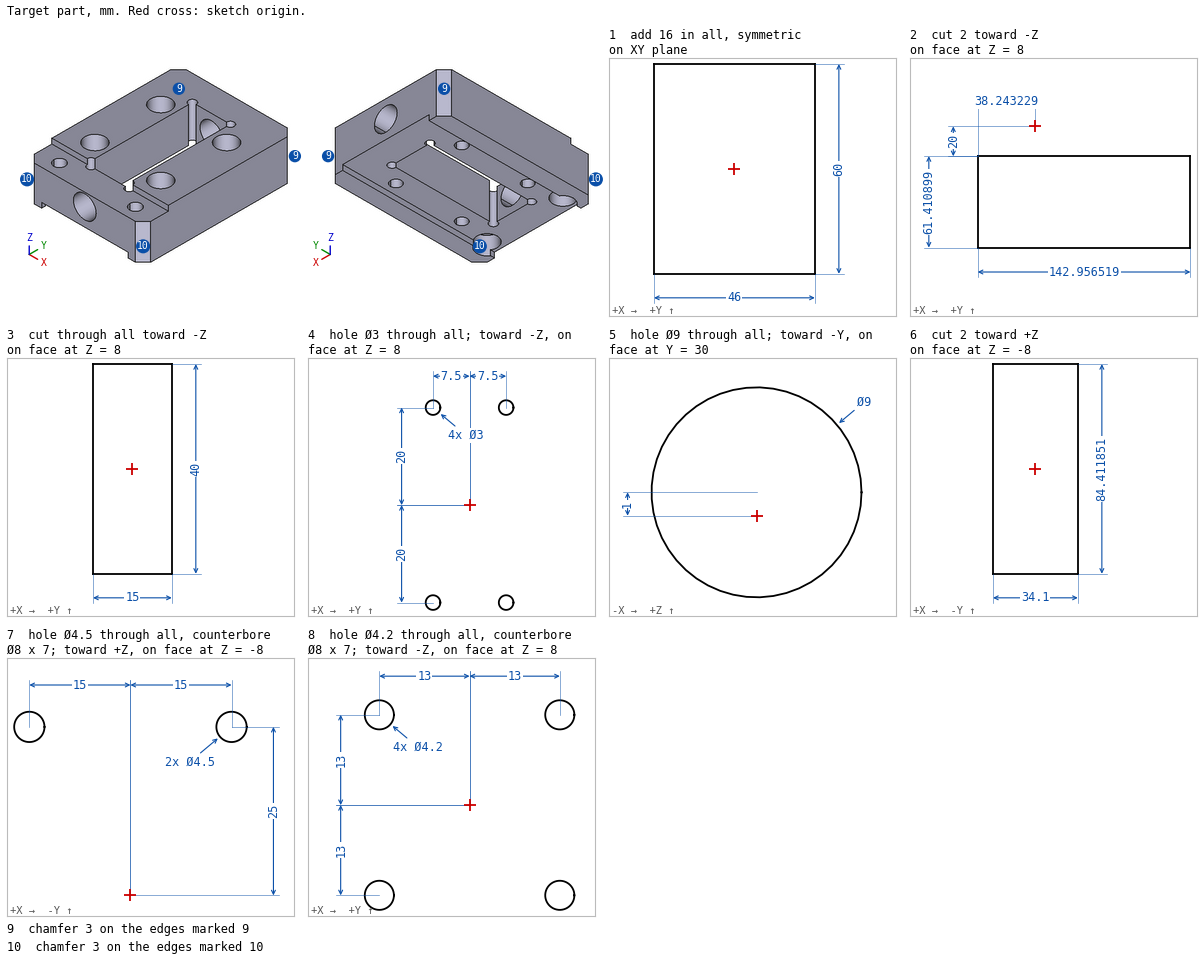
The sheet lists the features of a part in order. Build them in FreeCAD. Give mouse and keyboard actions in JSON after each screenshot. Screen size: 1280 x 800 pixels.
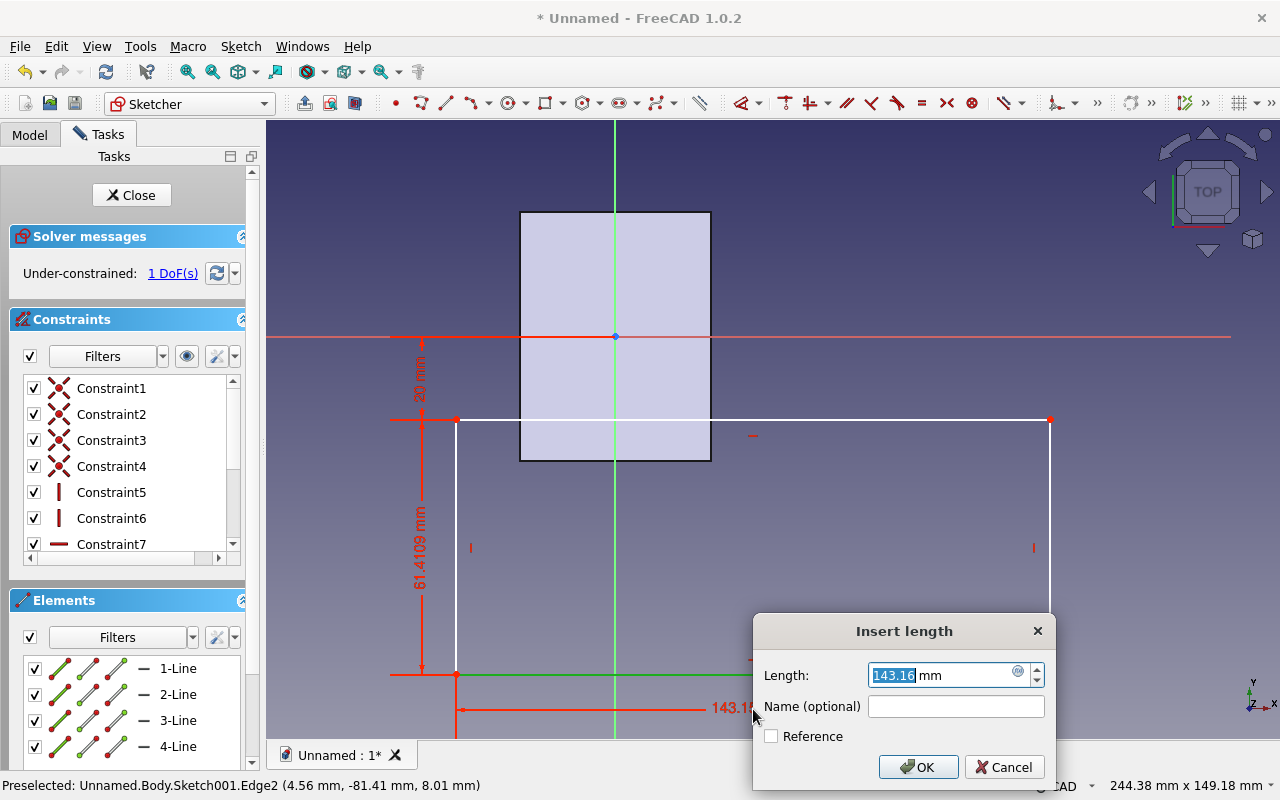
{"action": "type", "text": "142.956519"}
{"action": "key", "text": "Return"}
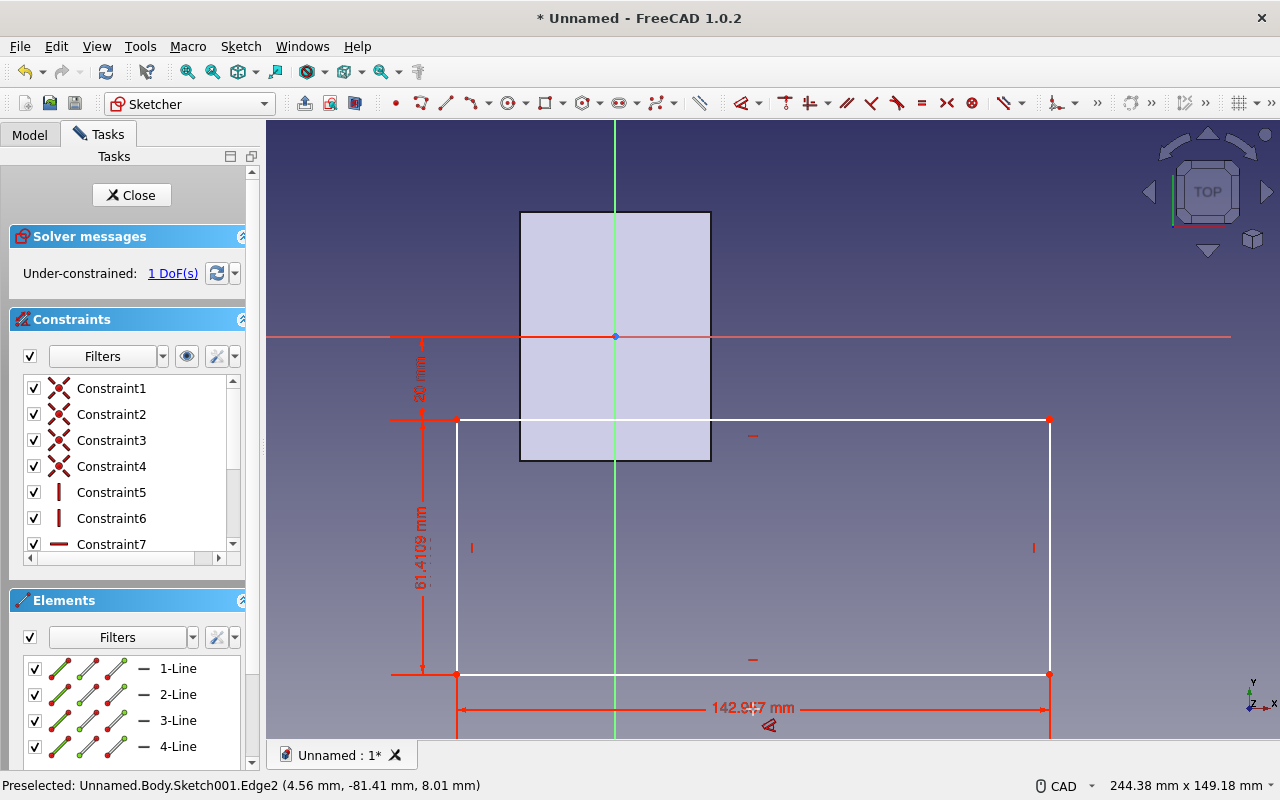
{"action": "left_click", "coordinate": [457, 420]}
{"action": "left_click", "coordinate": [536, 303]}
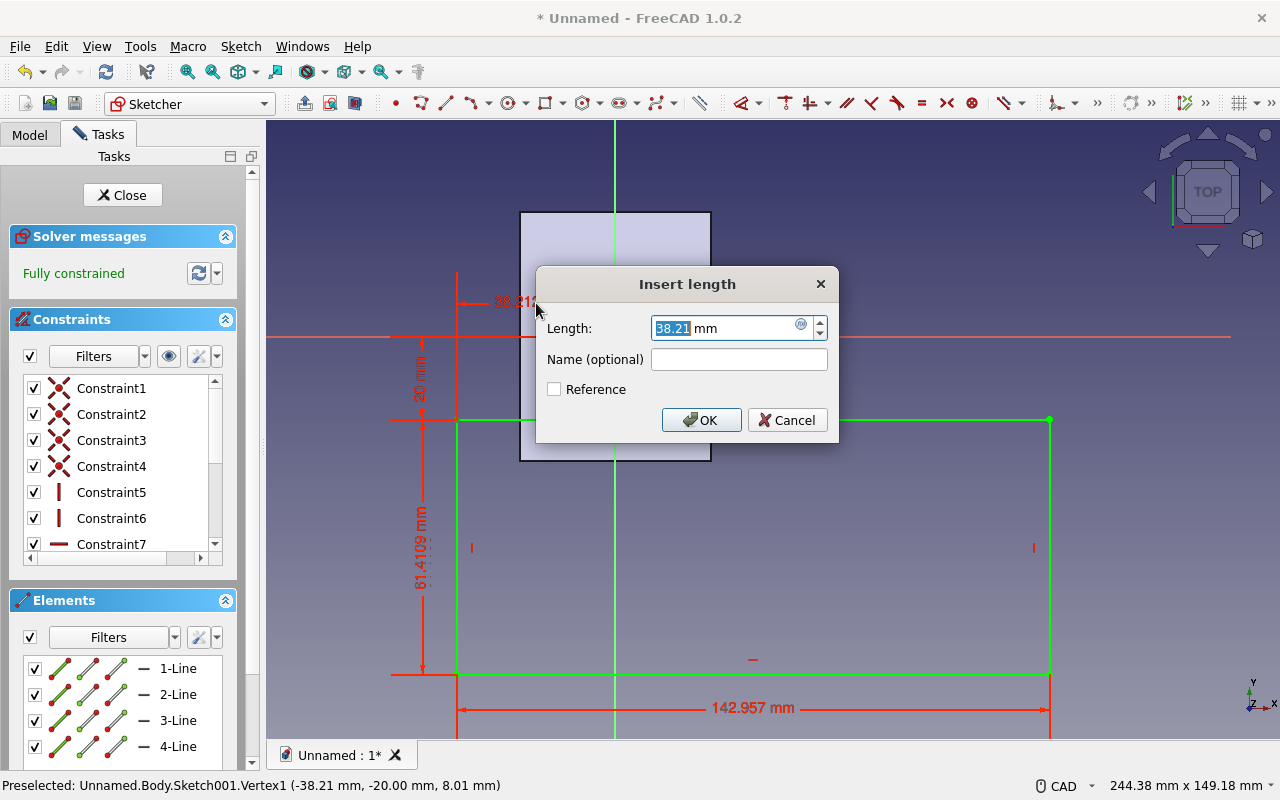
{"action": "type", "text": "38.243229"}
{"action": "key", "text": "Return"}
{"action": "key", "text": "Escape"}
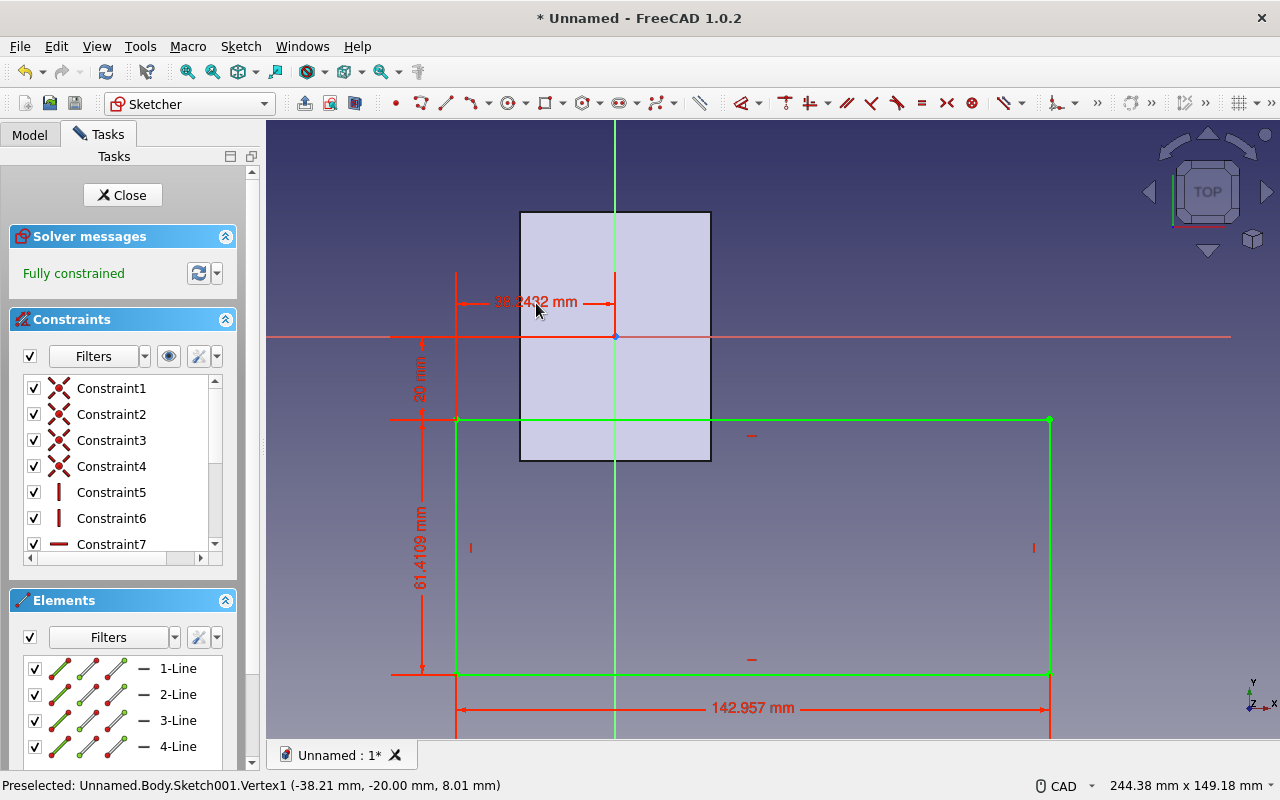
{"action": "left_click", "coordinate": [123, 195]}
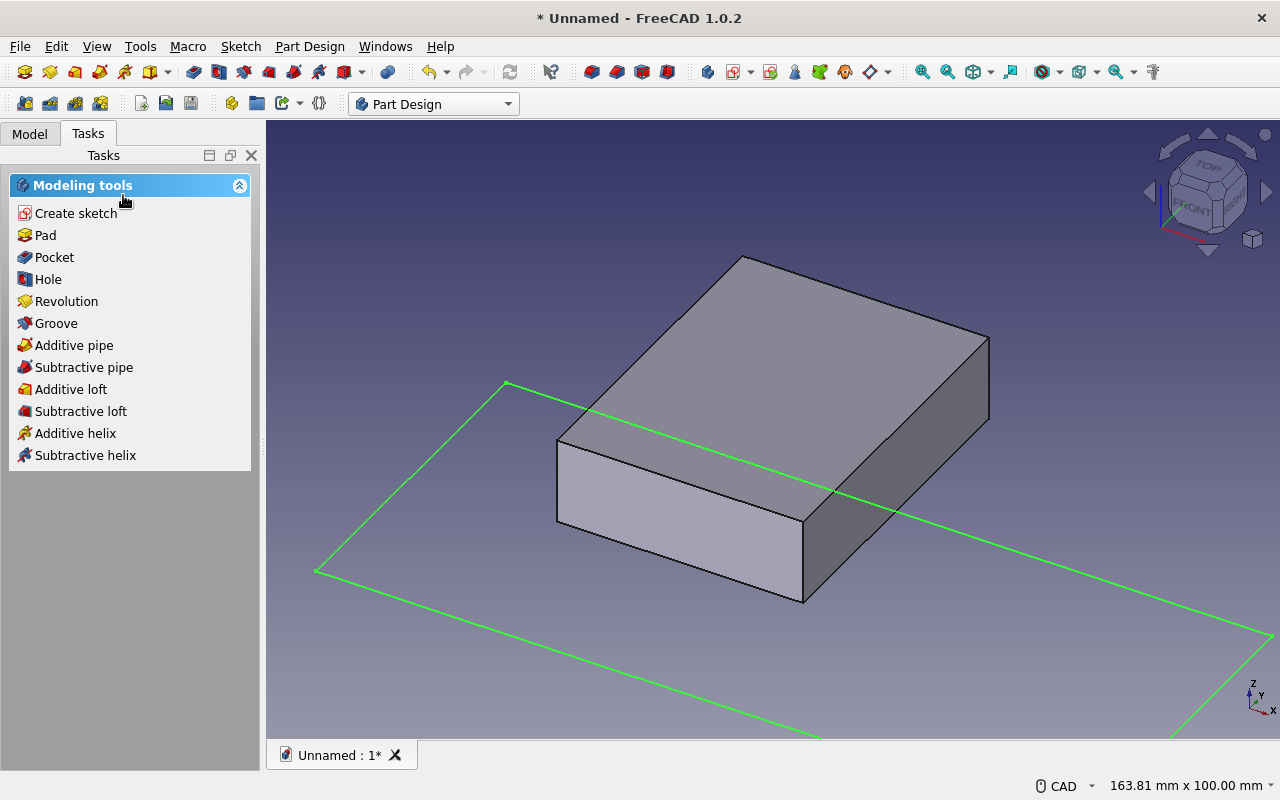
{"action": "left_click", "coordinate": [194, 72]}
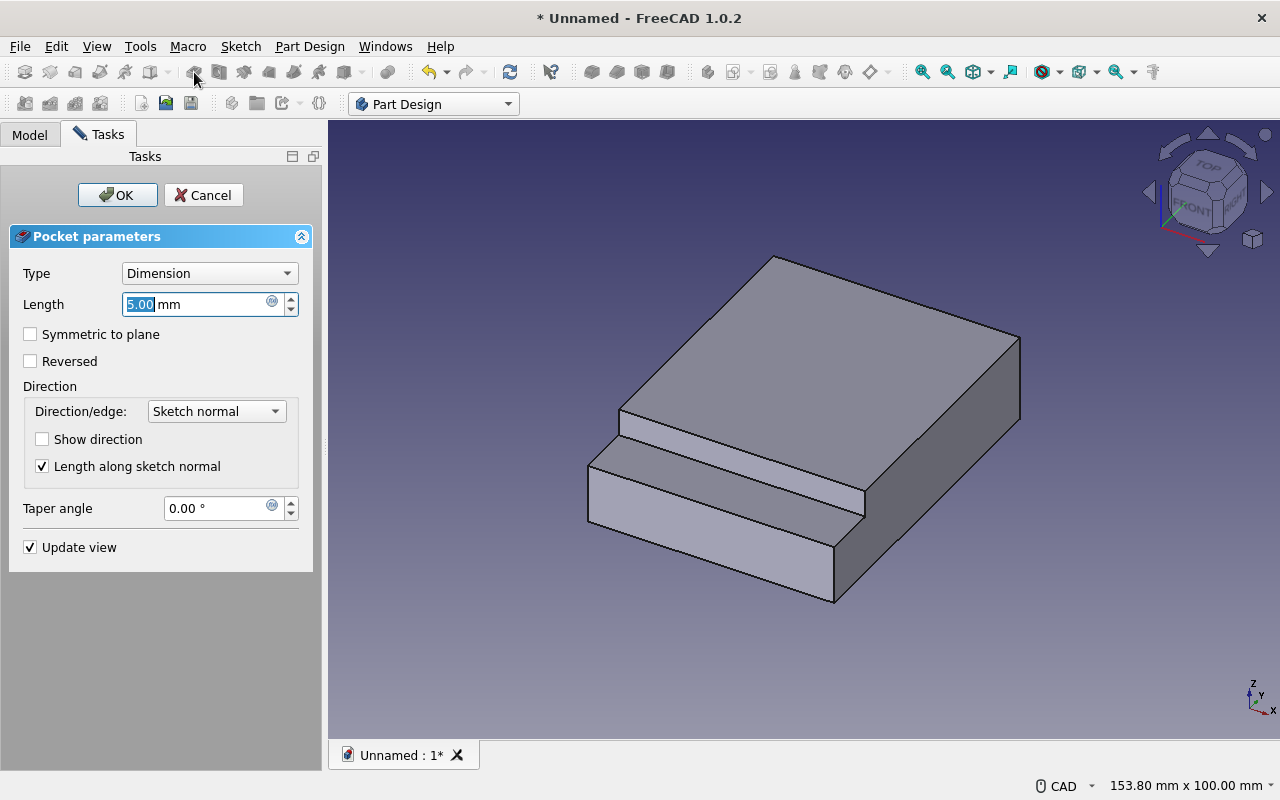
{"action": "type", "text": "2"}
{"action": "key", "text": "Tab"}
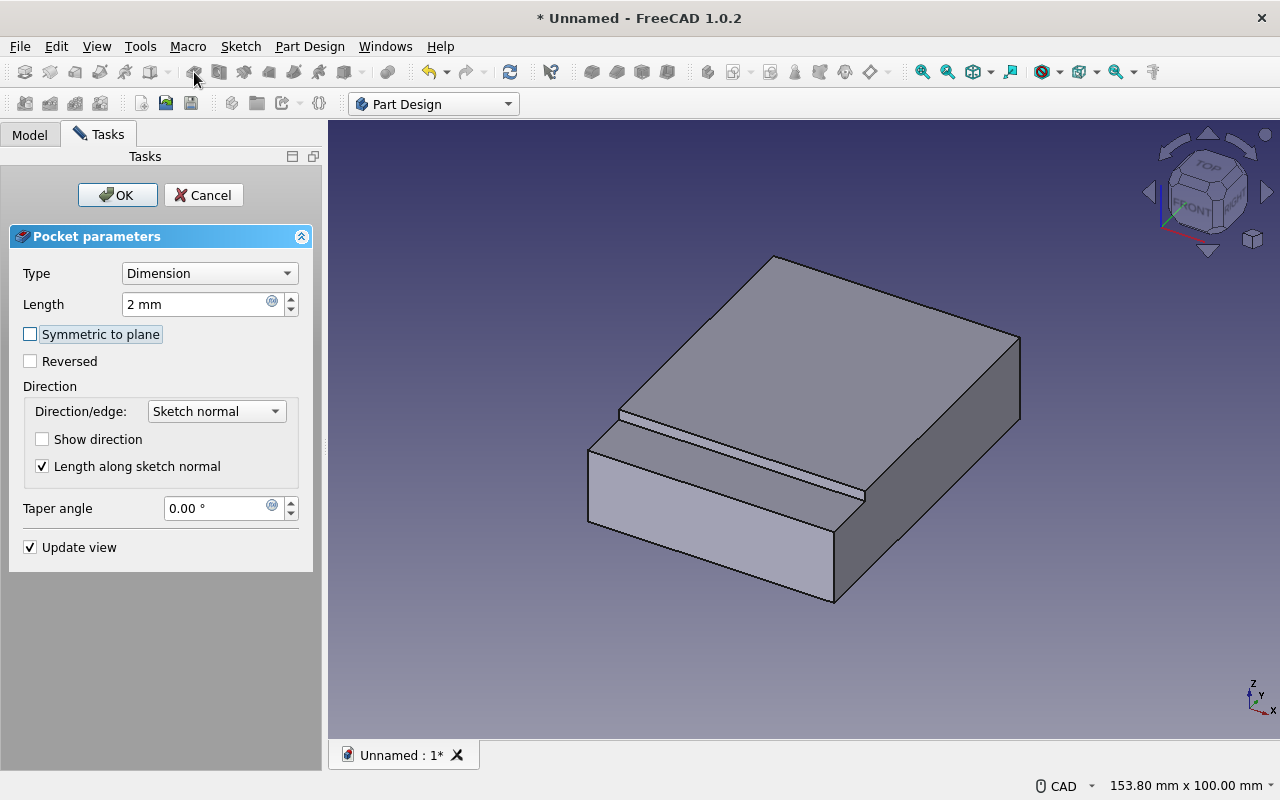
{"action": "left_click", "coordinate": [118, 195]}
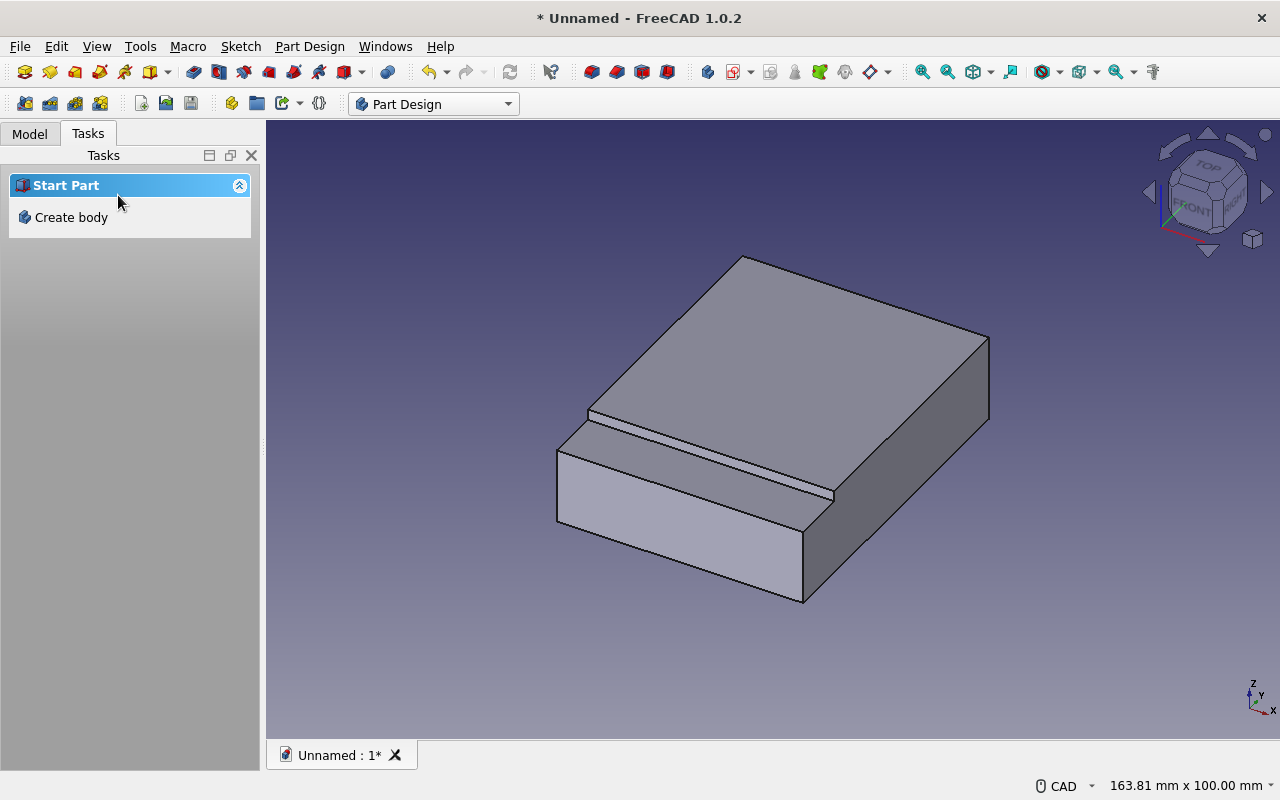
{"action": "left_click", "coordinate": [788, 373]}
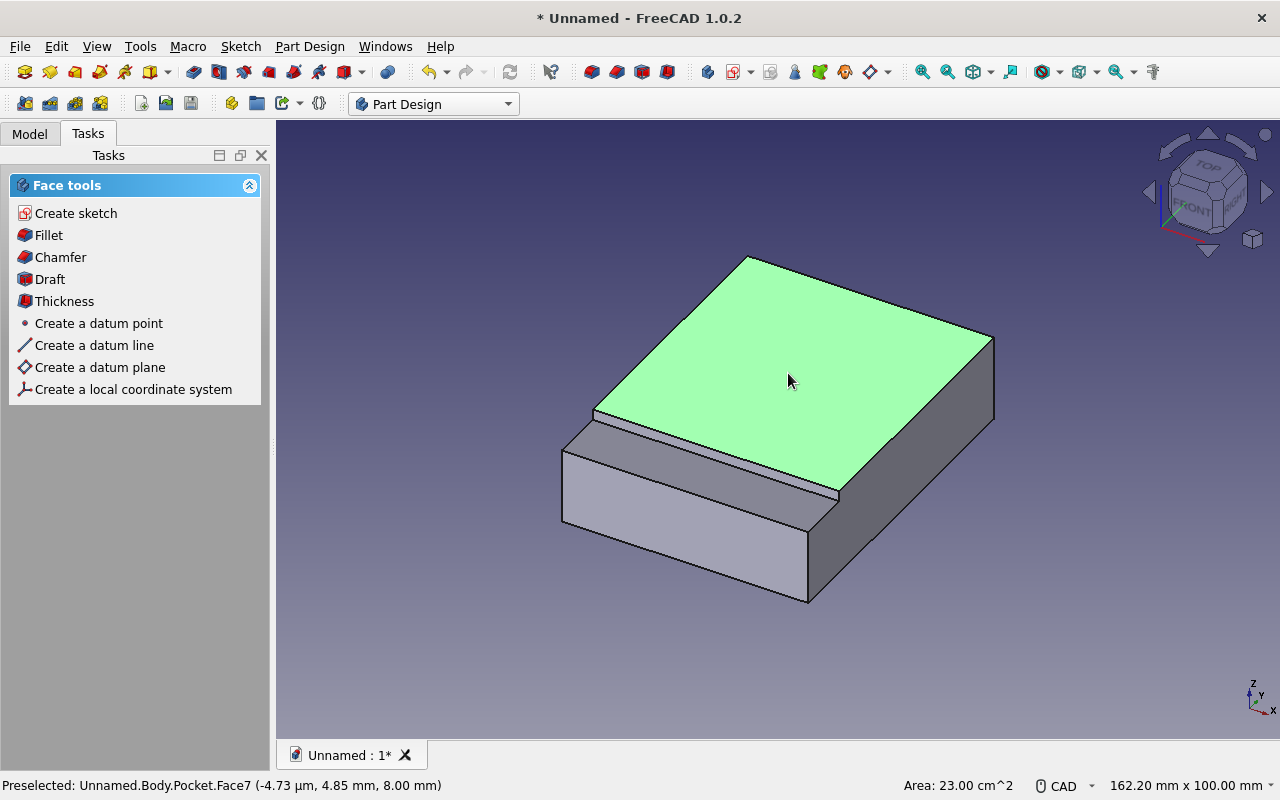
{"action": "left_click", "coordinate": [732, 72]}